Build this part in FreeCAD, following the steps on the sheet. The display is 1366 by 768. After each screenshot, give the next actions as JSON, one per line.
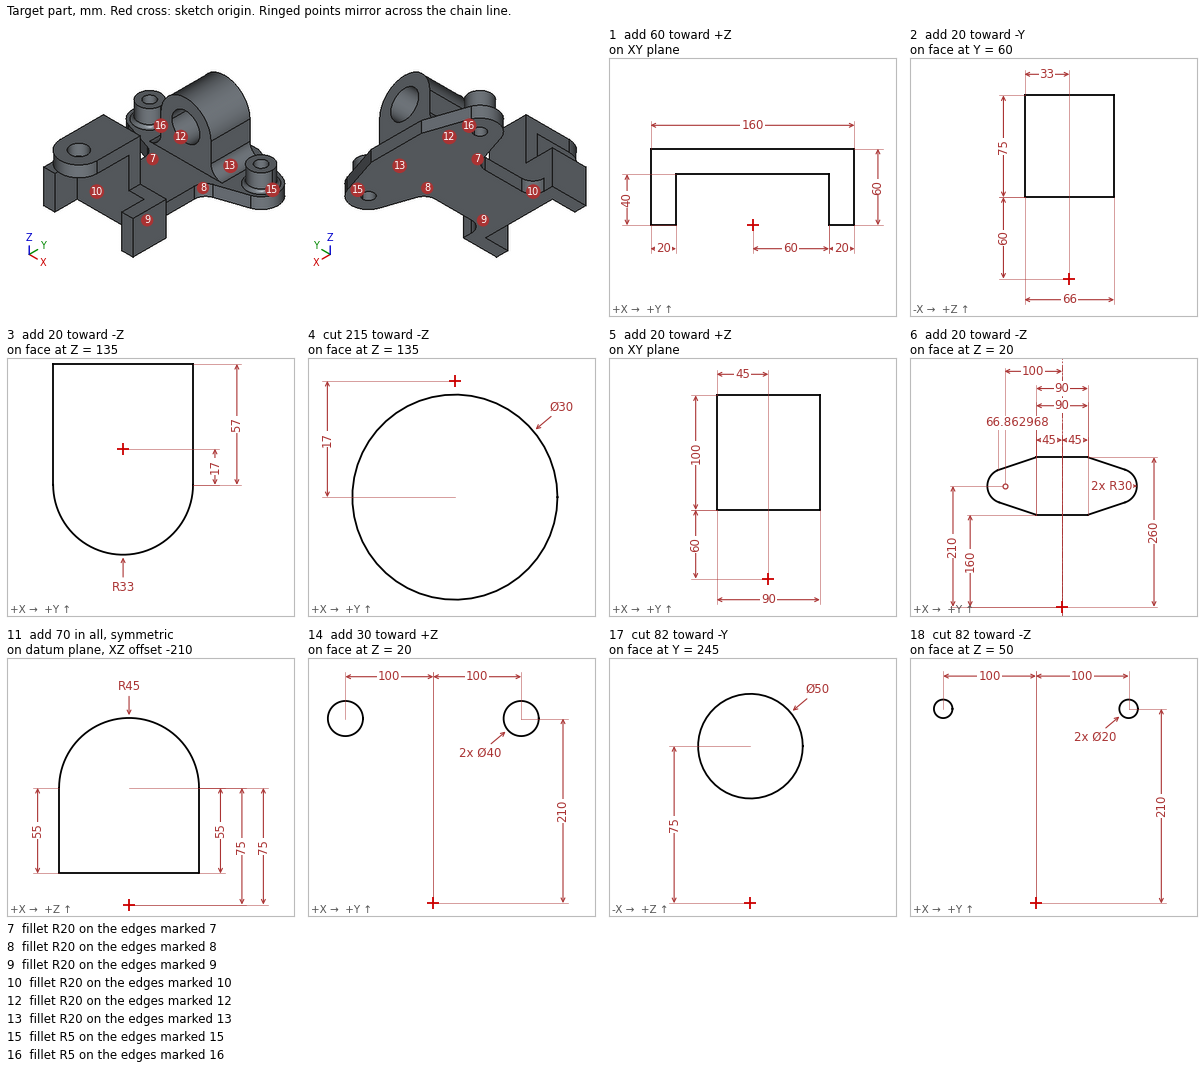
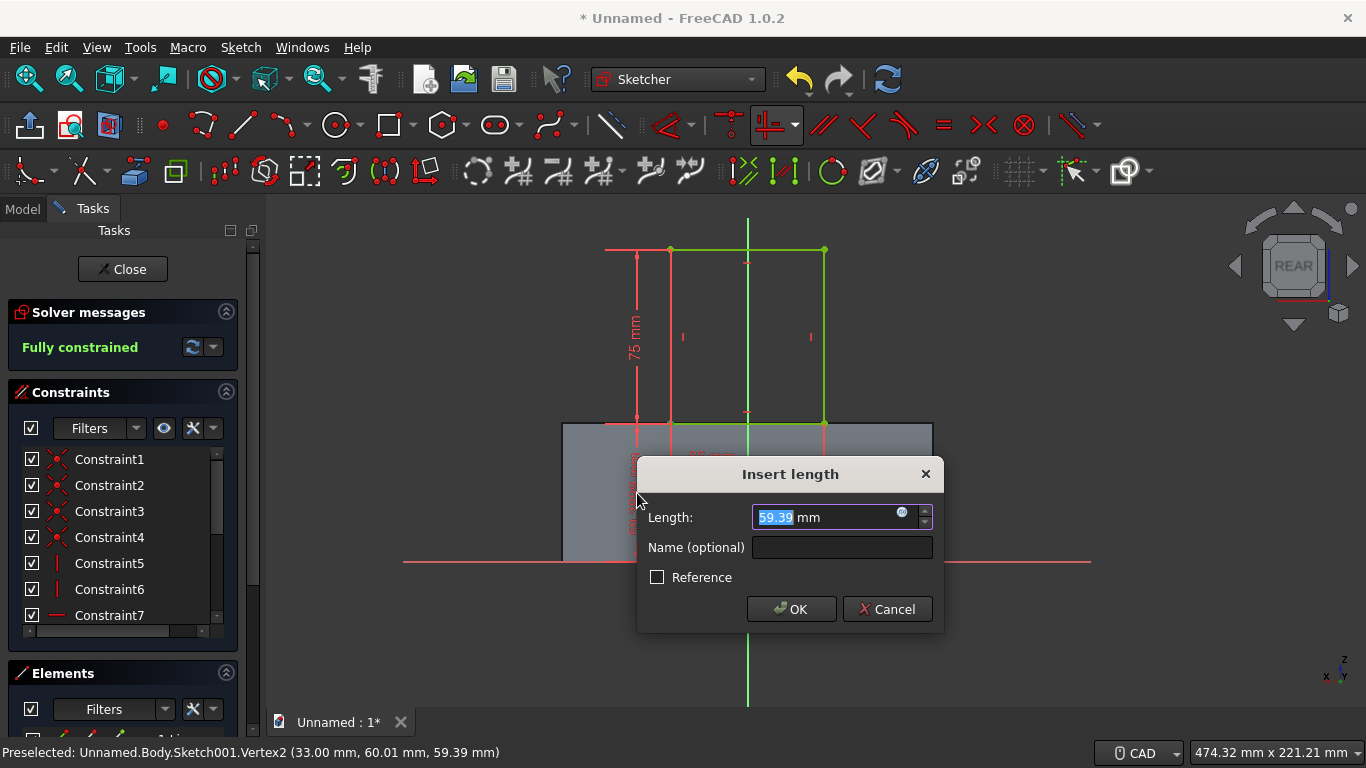
{"action": "type", "text": "60"}
{"action": "key", "text": "Return"}
{"action": "key", "text": "Escape"}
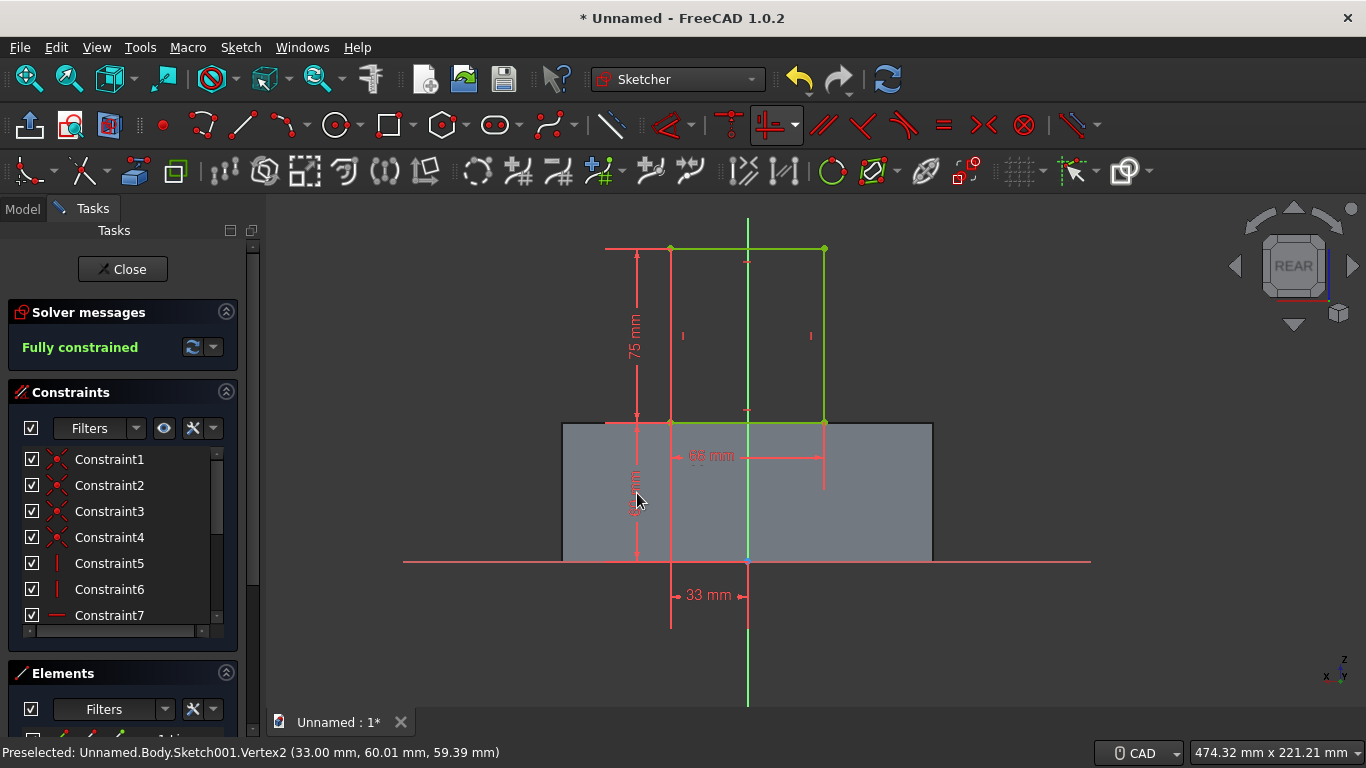
{"action": "left_click", "coordinate": [123, 269]}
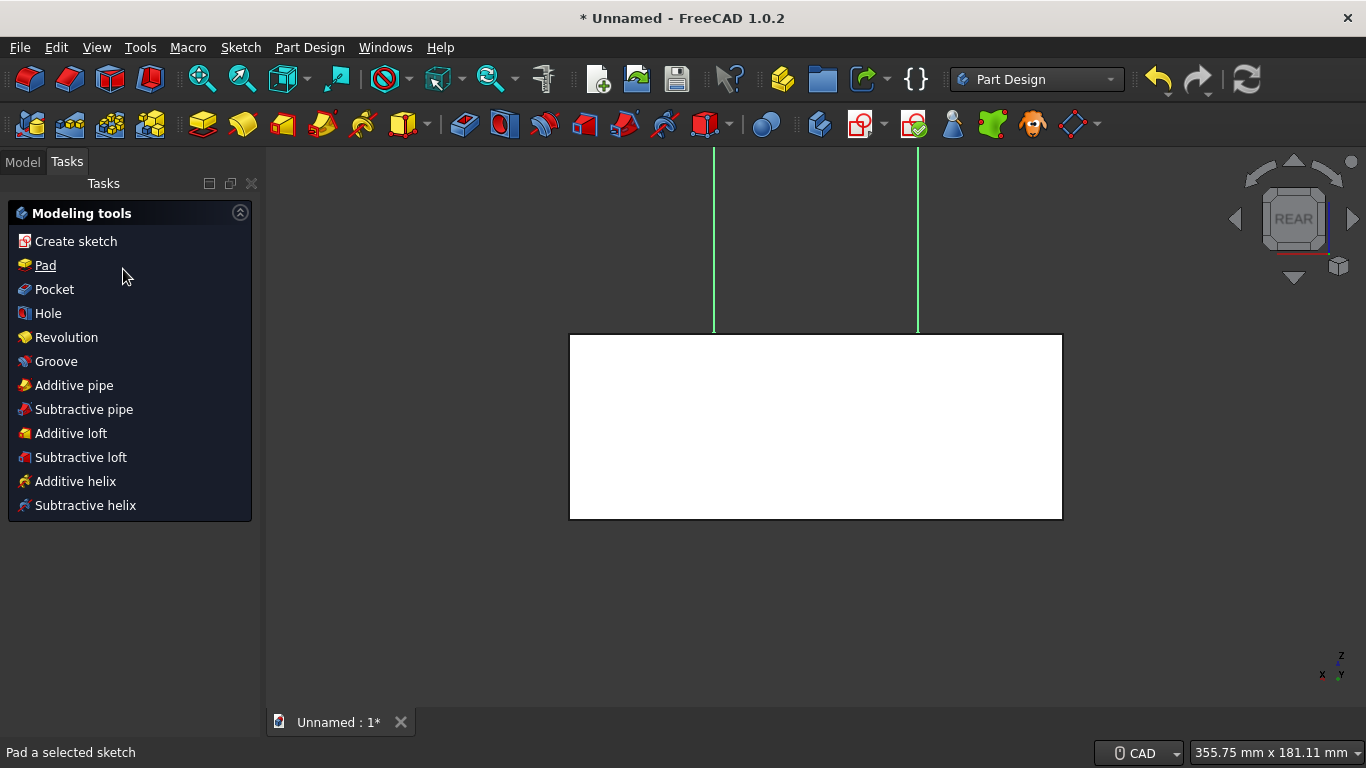
{"action": "left_click", "coordinate": [204, 124]}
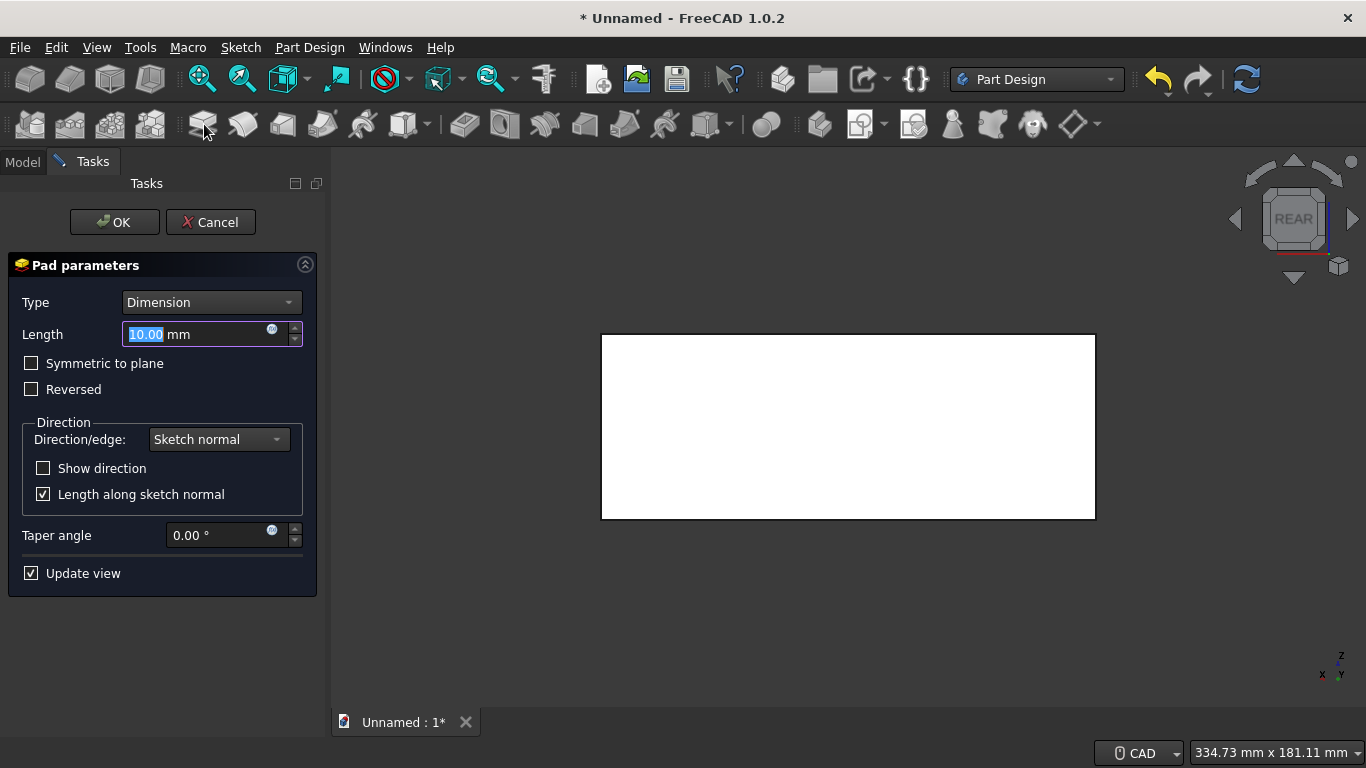
{"action": "type", "text": "20"}
{"action": "key", "text": "Tab"}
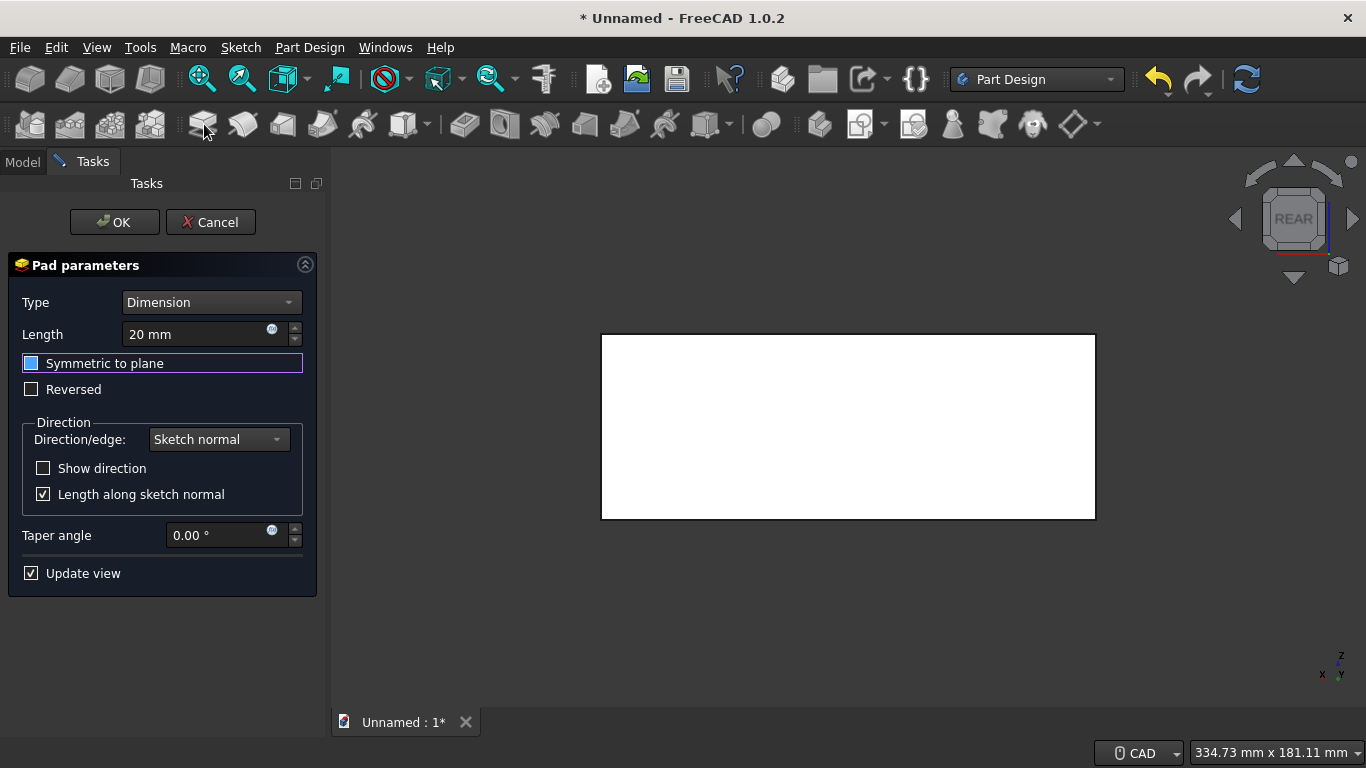
{"action": "left_click", "coordinate": [30, 389]}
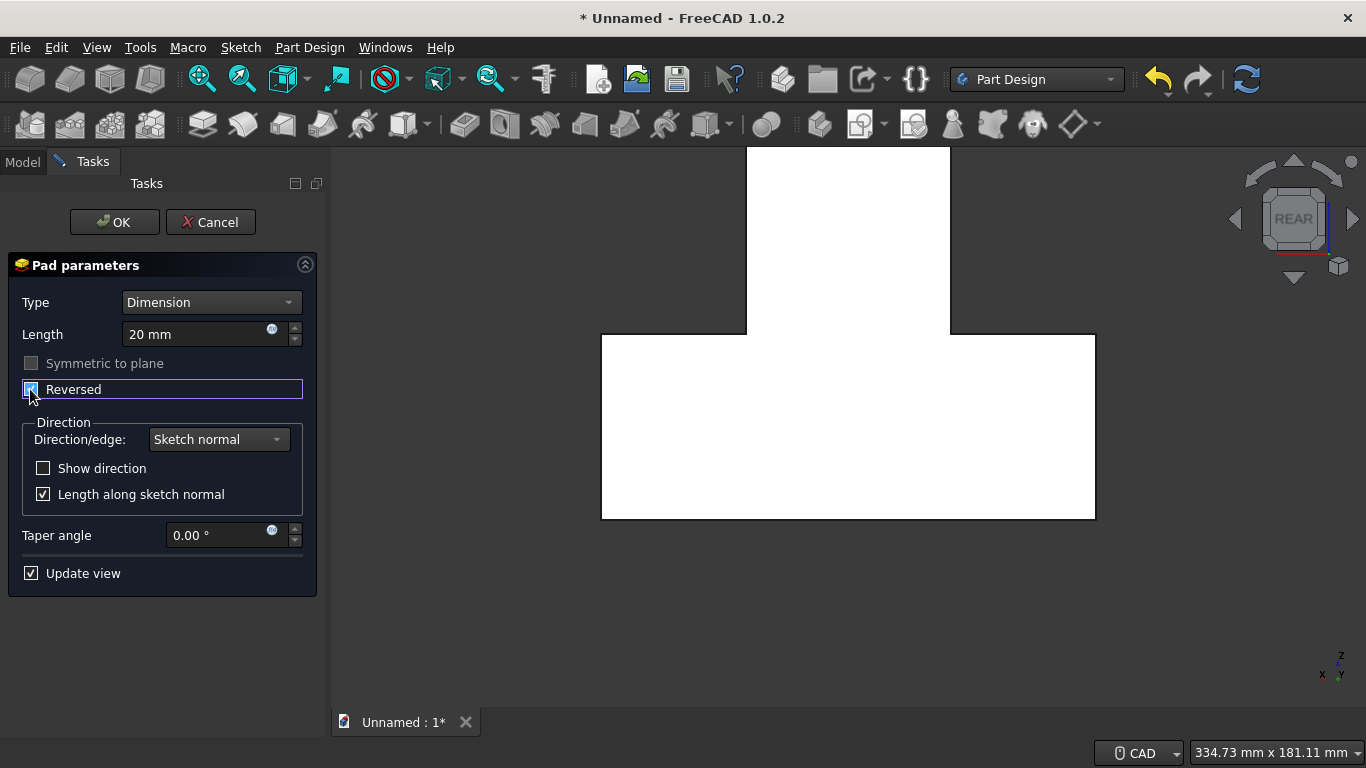
{"action": "left_click", "coordinate": [115, 222]}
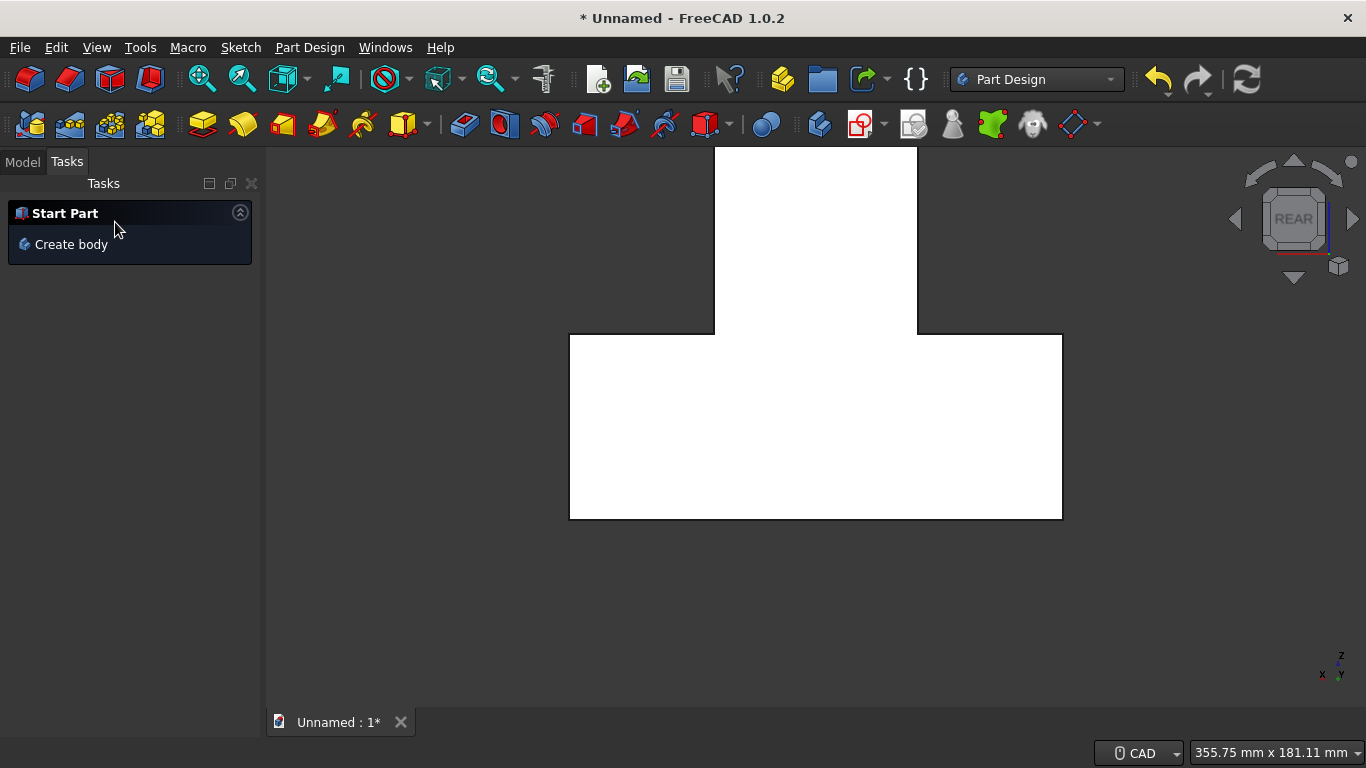
{"action": "key", "text": "v f"}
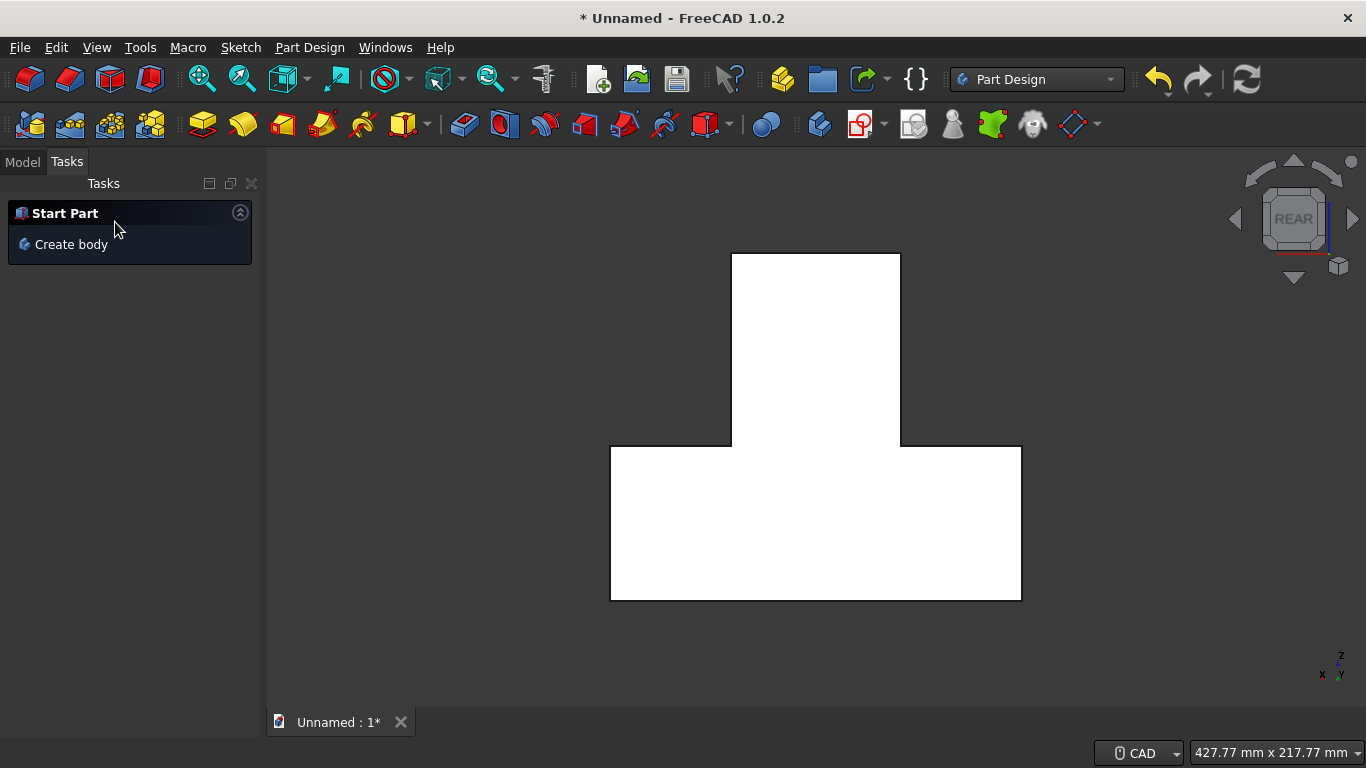
{"action": "key", "text": "0"}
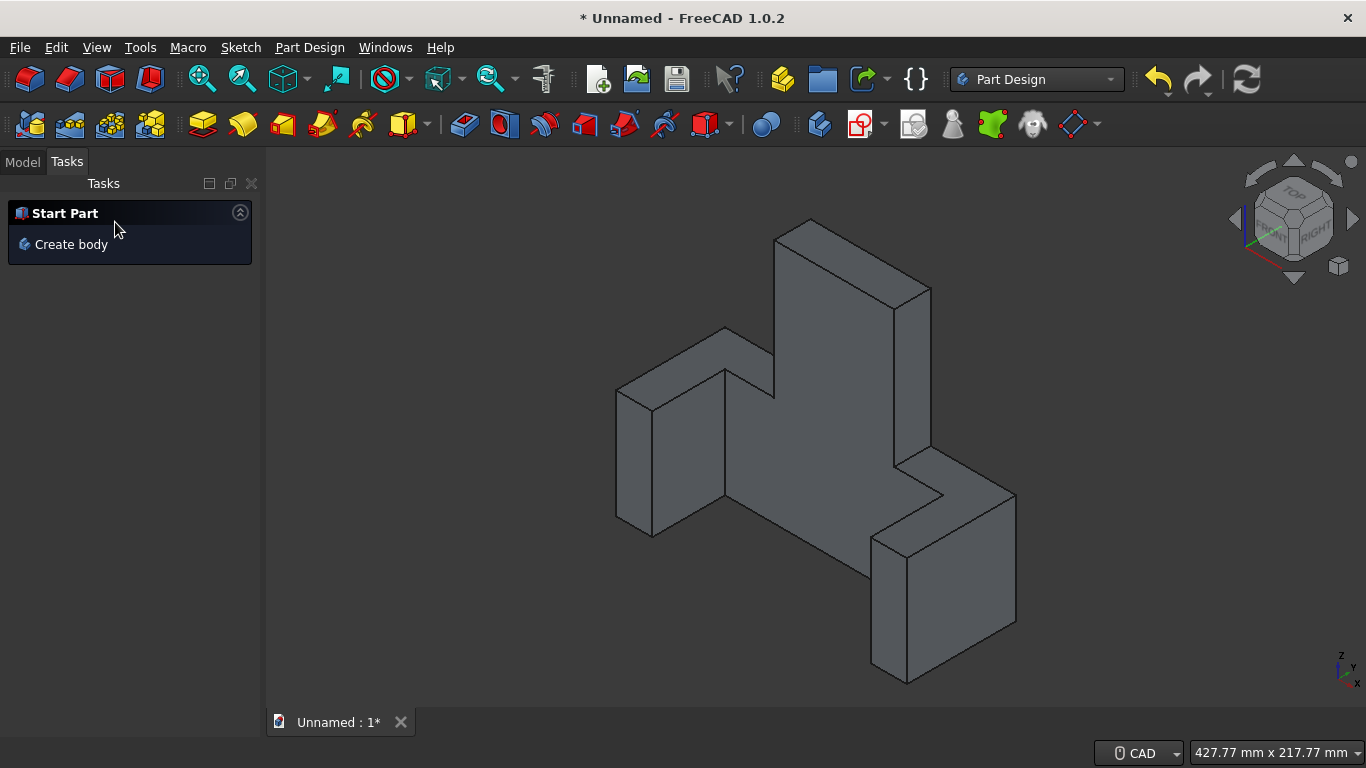
{"action": "left_click", "coordinate": [887, 283]}